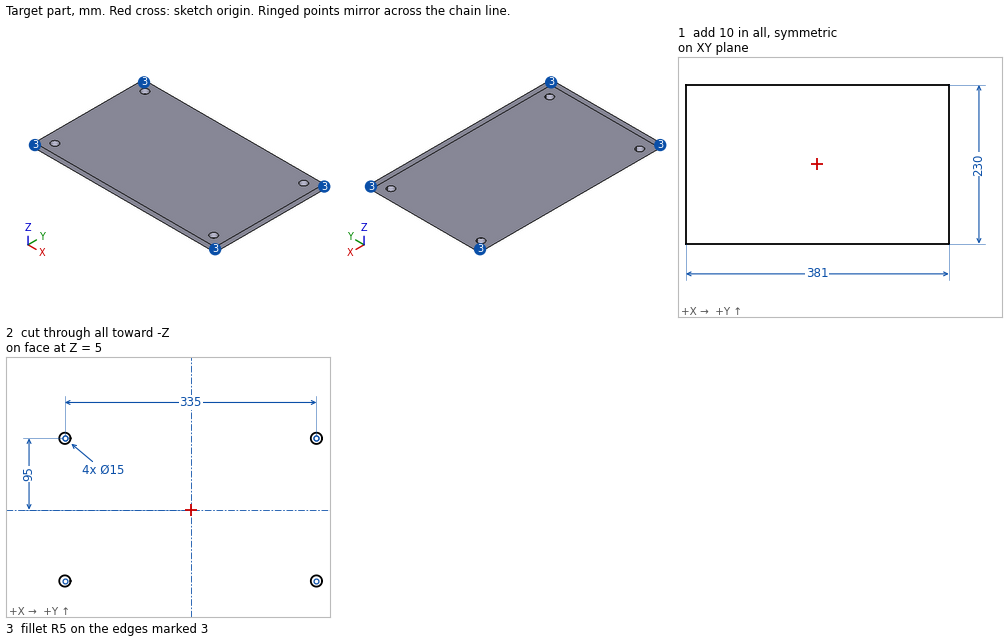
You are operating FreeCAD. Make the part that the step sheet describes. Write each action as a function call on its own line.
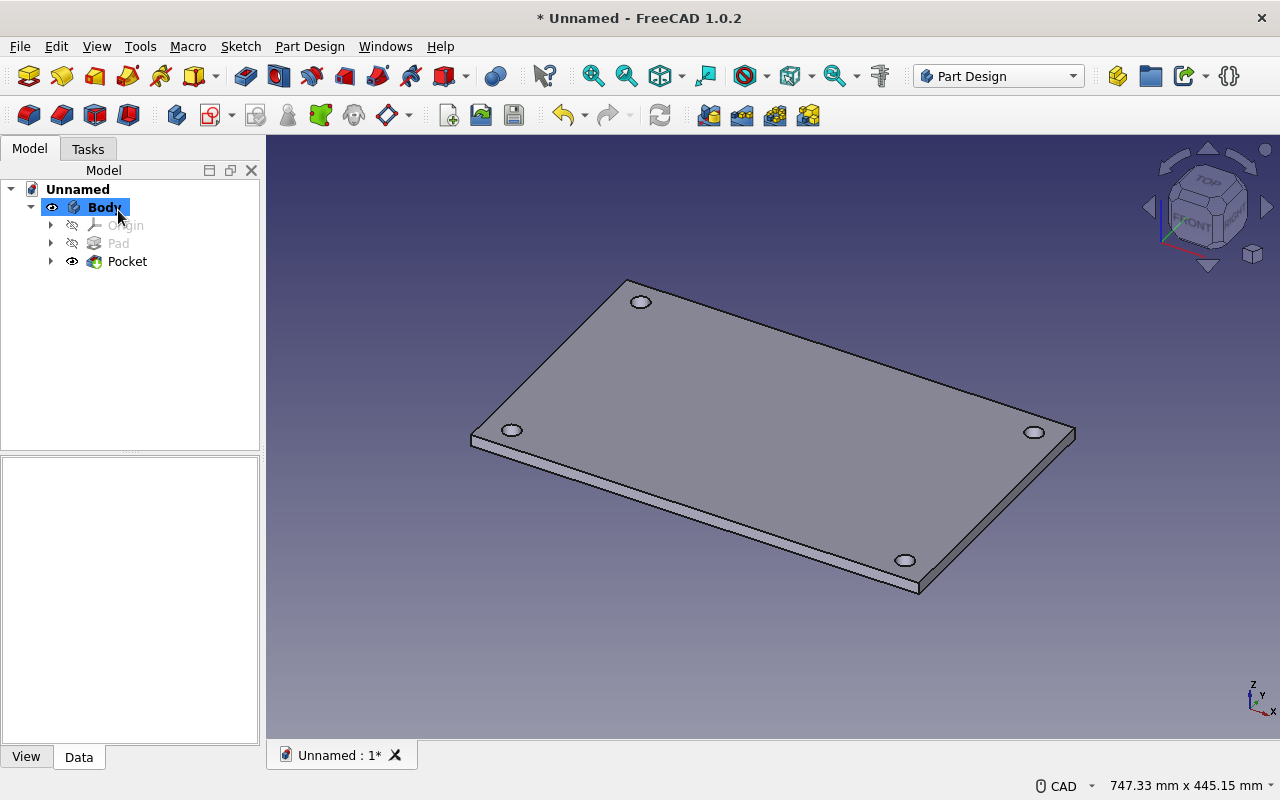
click(919, 589)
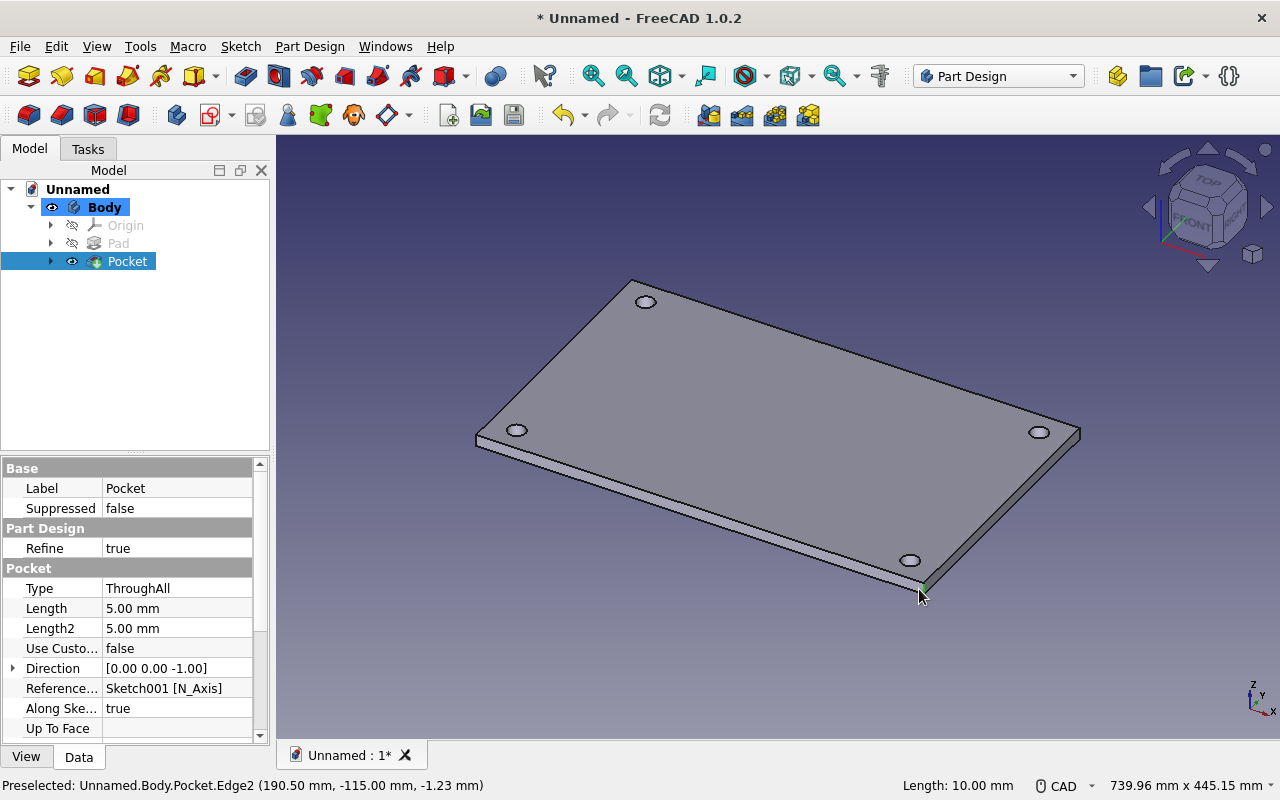
scroll(632, 284, up, 6)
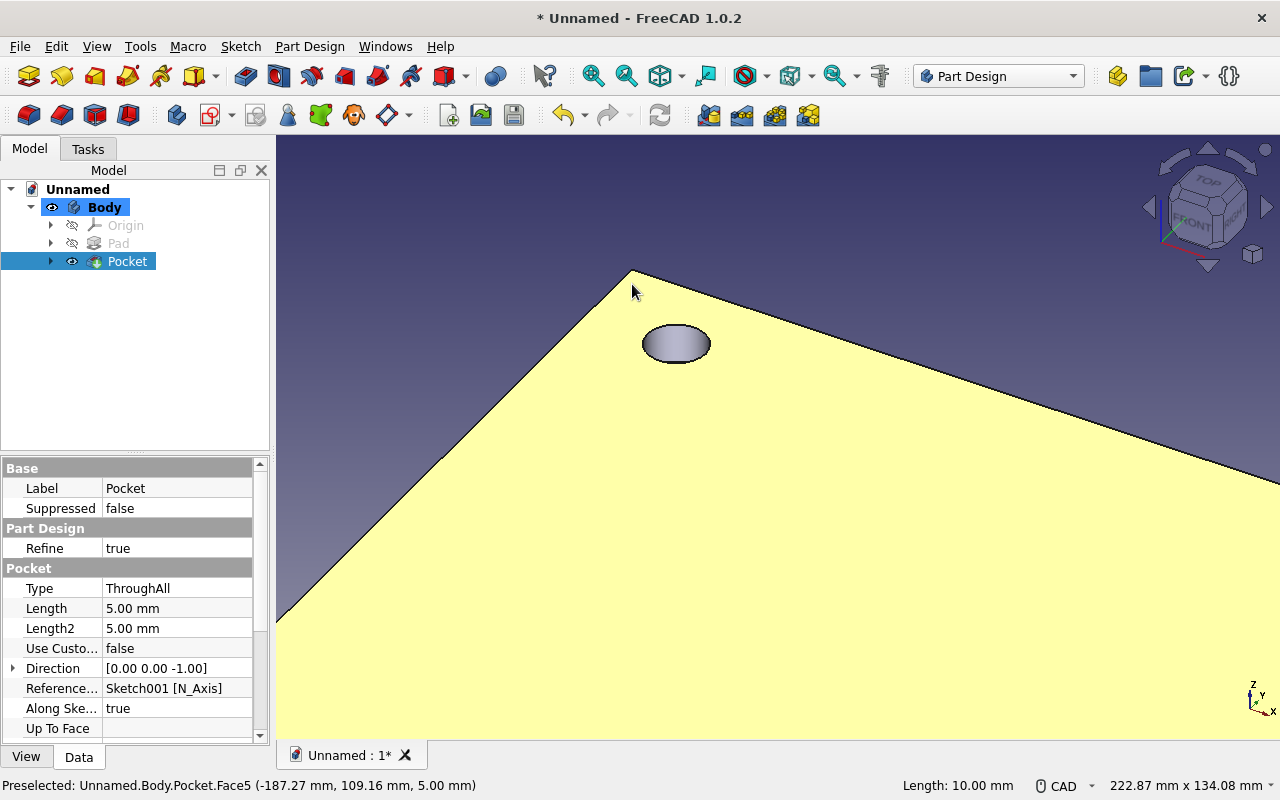
click(594, 76)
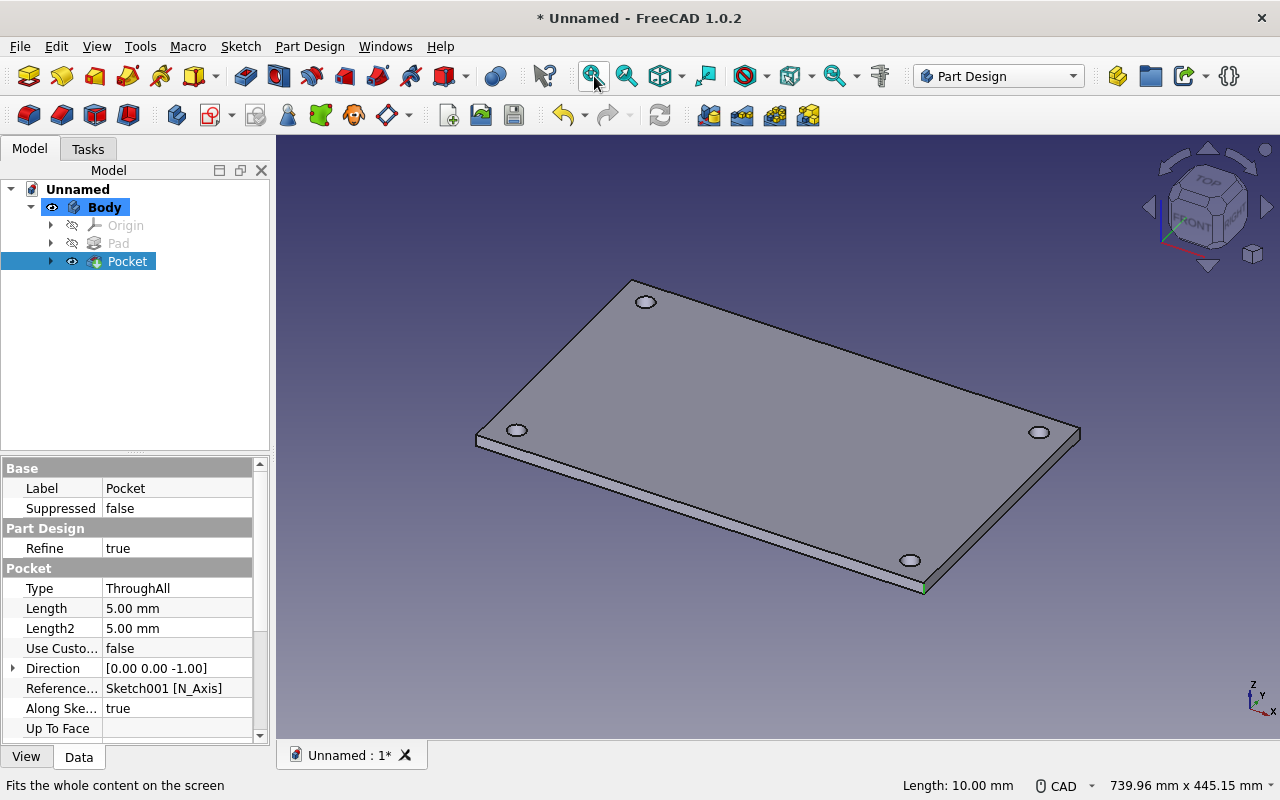
key(0)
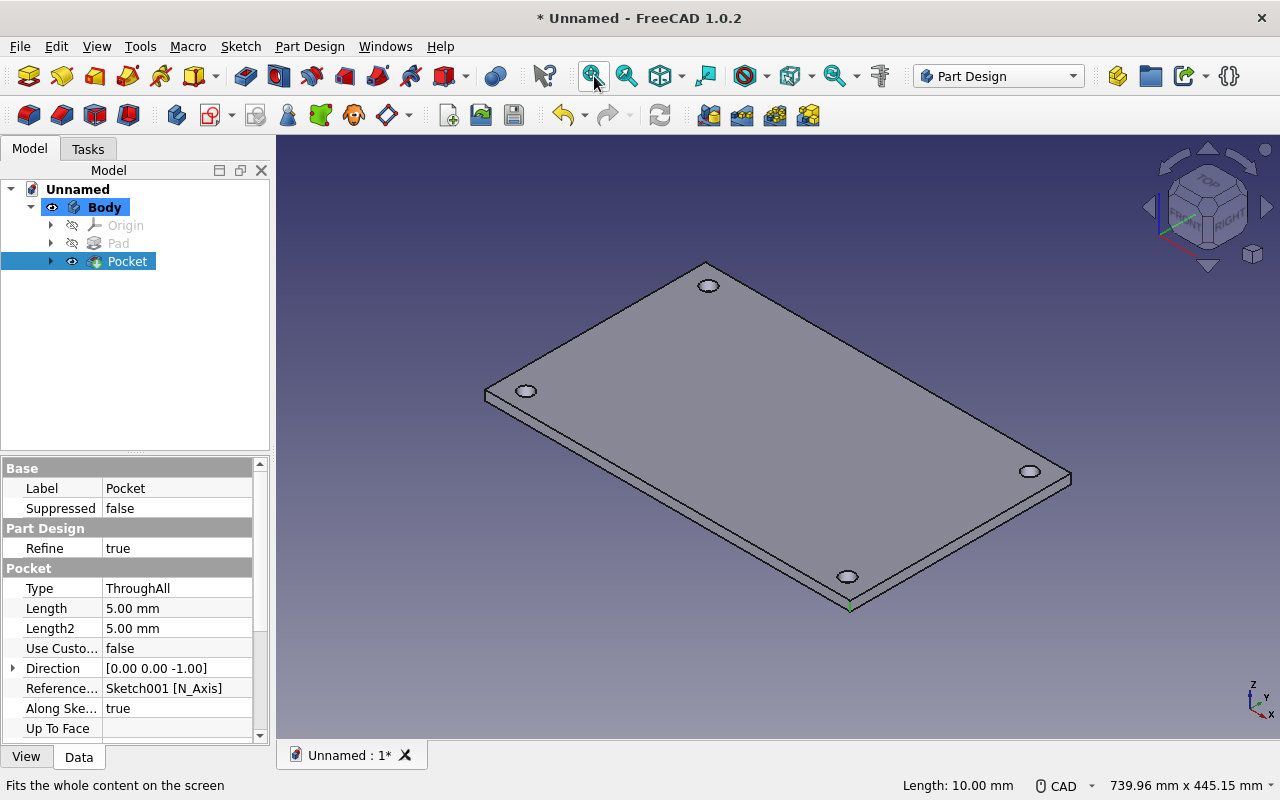
scroll(706, 267, up, 6)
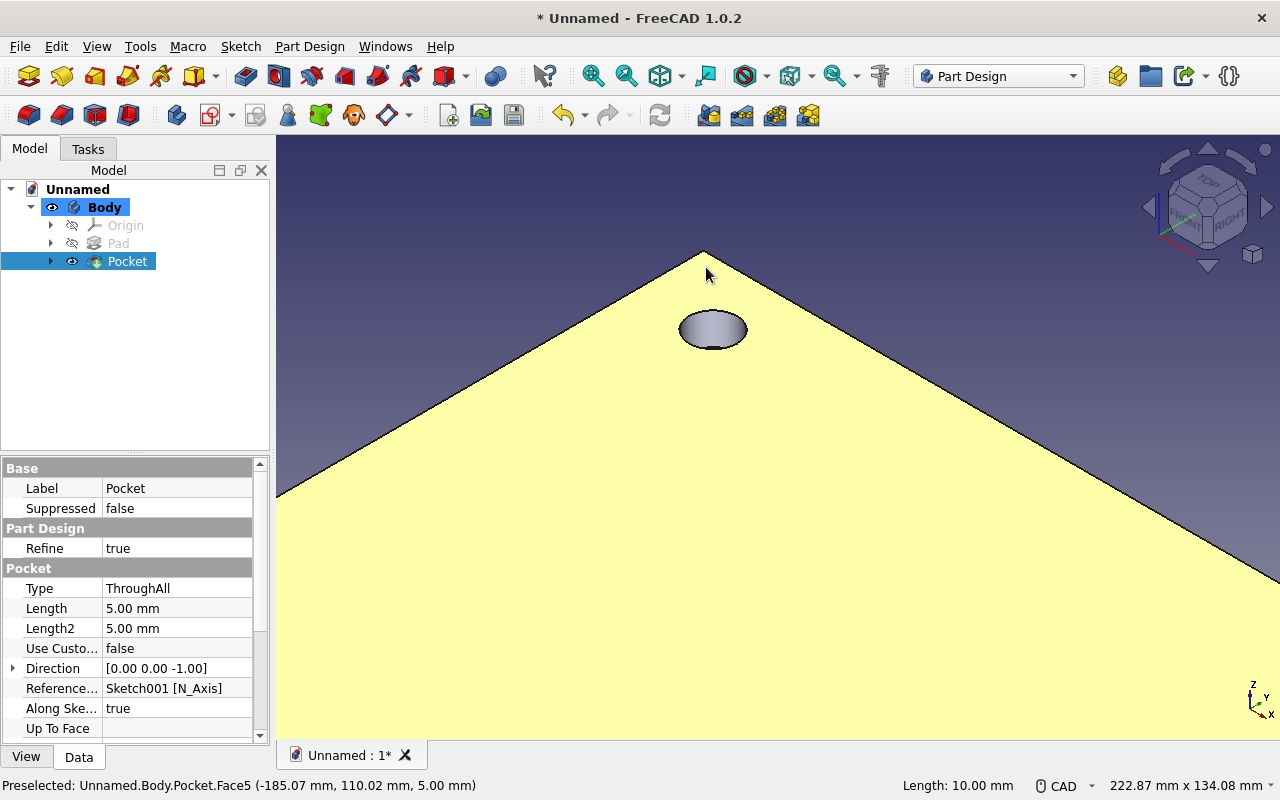
key(v)
key(f)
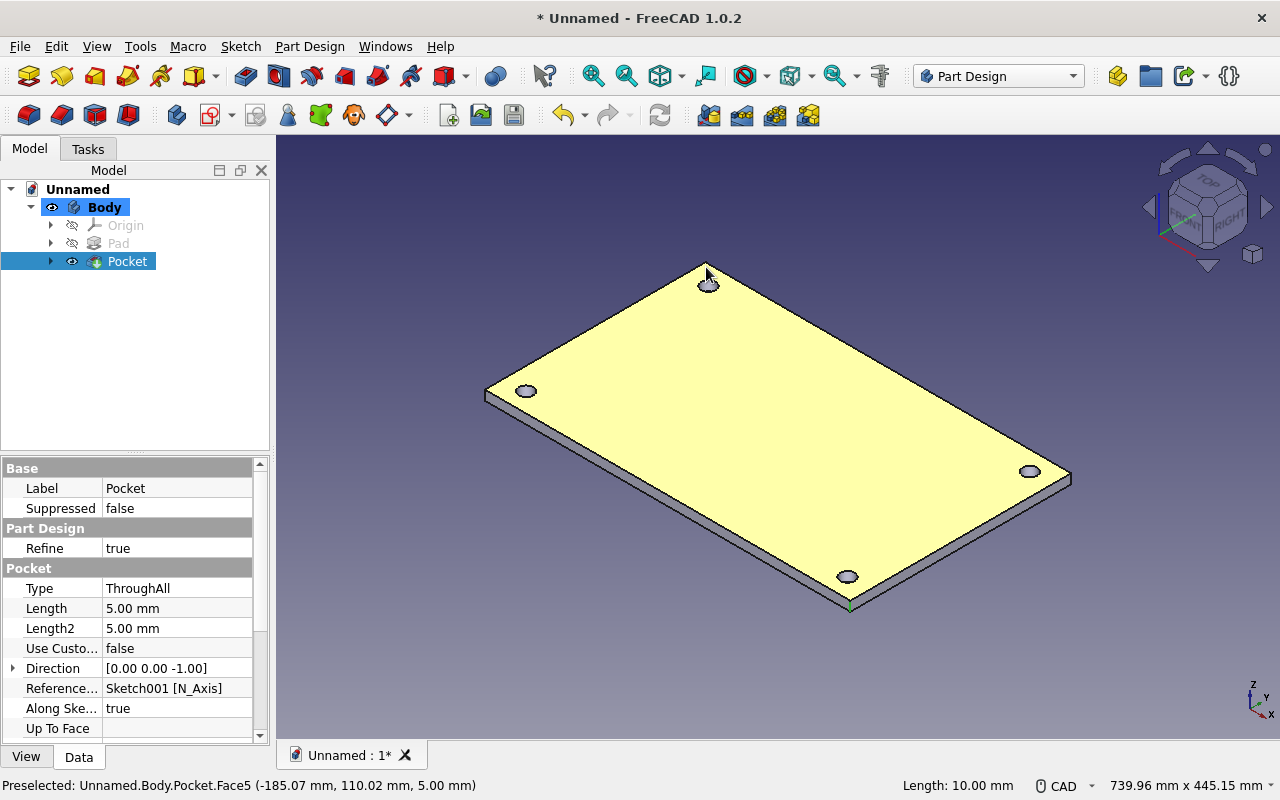
key(2)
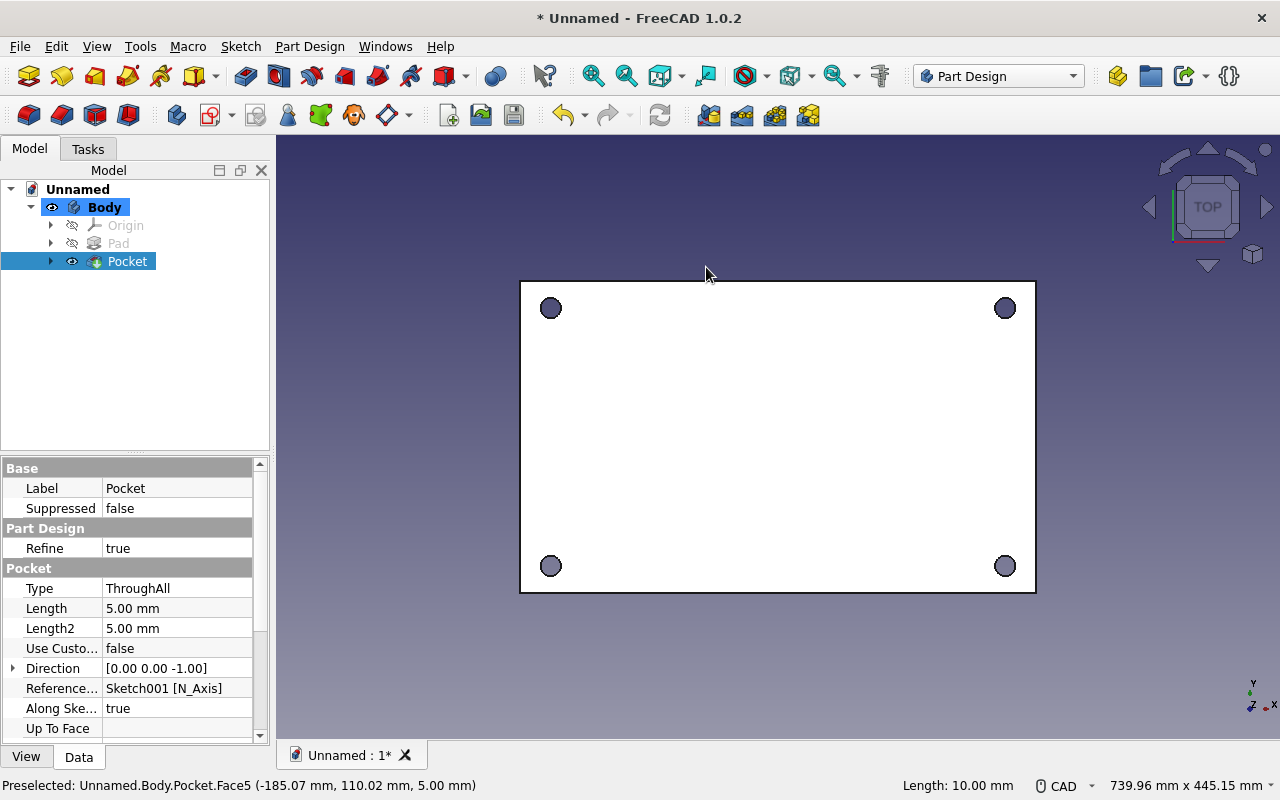
scroll(520, 280, up, 6)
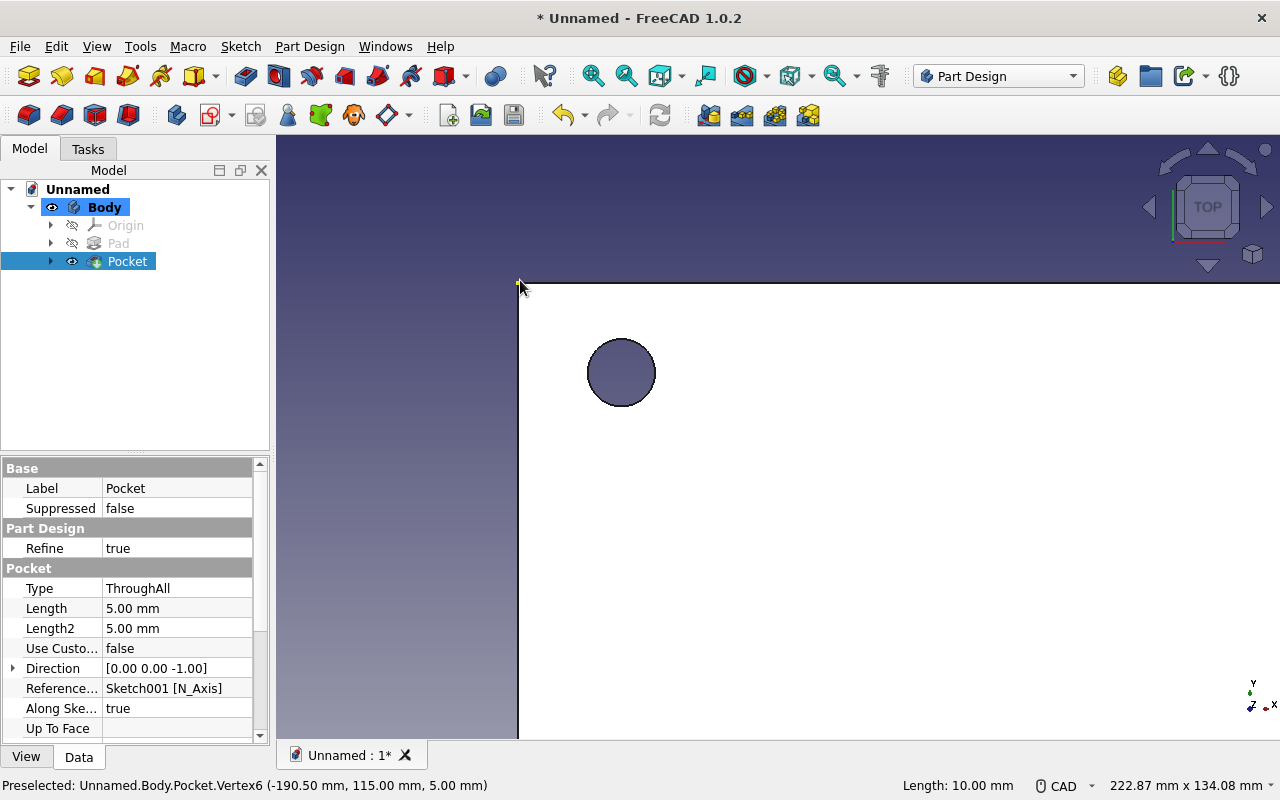
click(594, 76)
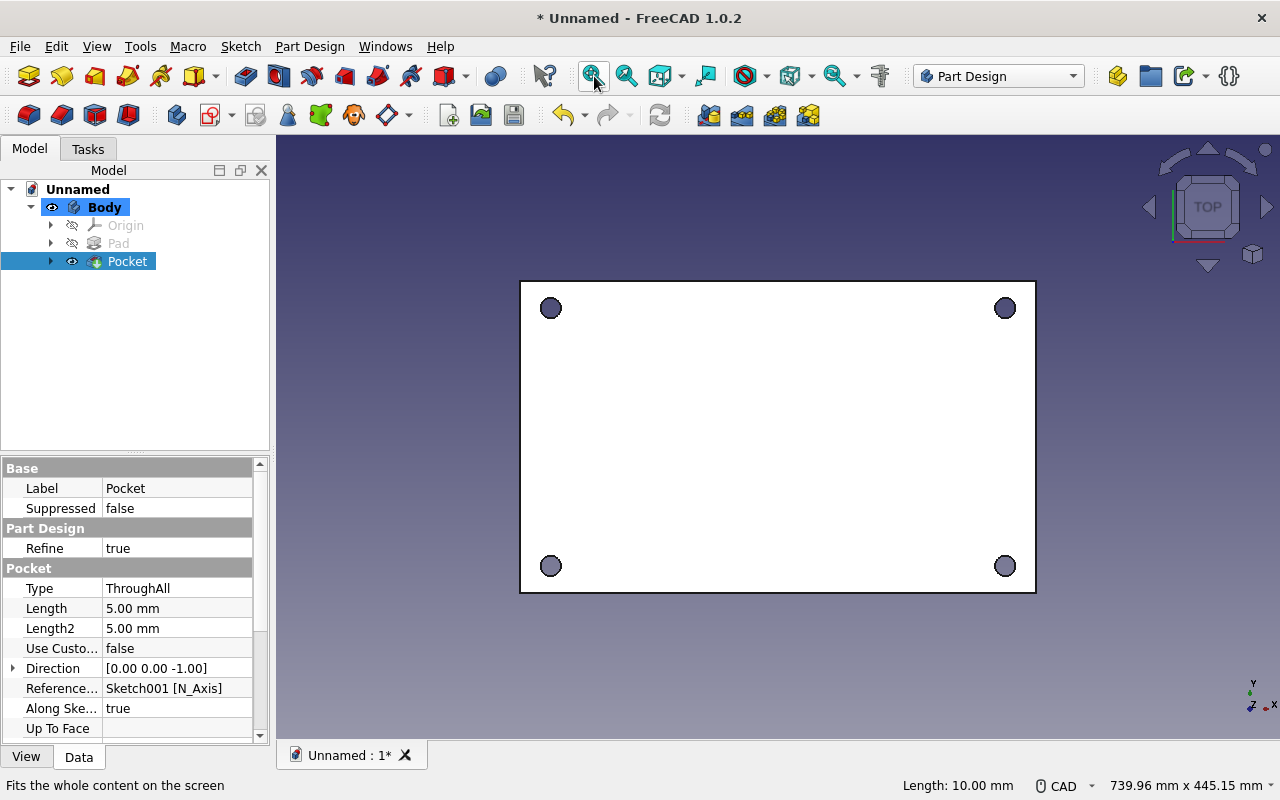
key(1)